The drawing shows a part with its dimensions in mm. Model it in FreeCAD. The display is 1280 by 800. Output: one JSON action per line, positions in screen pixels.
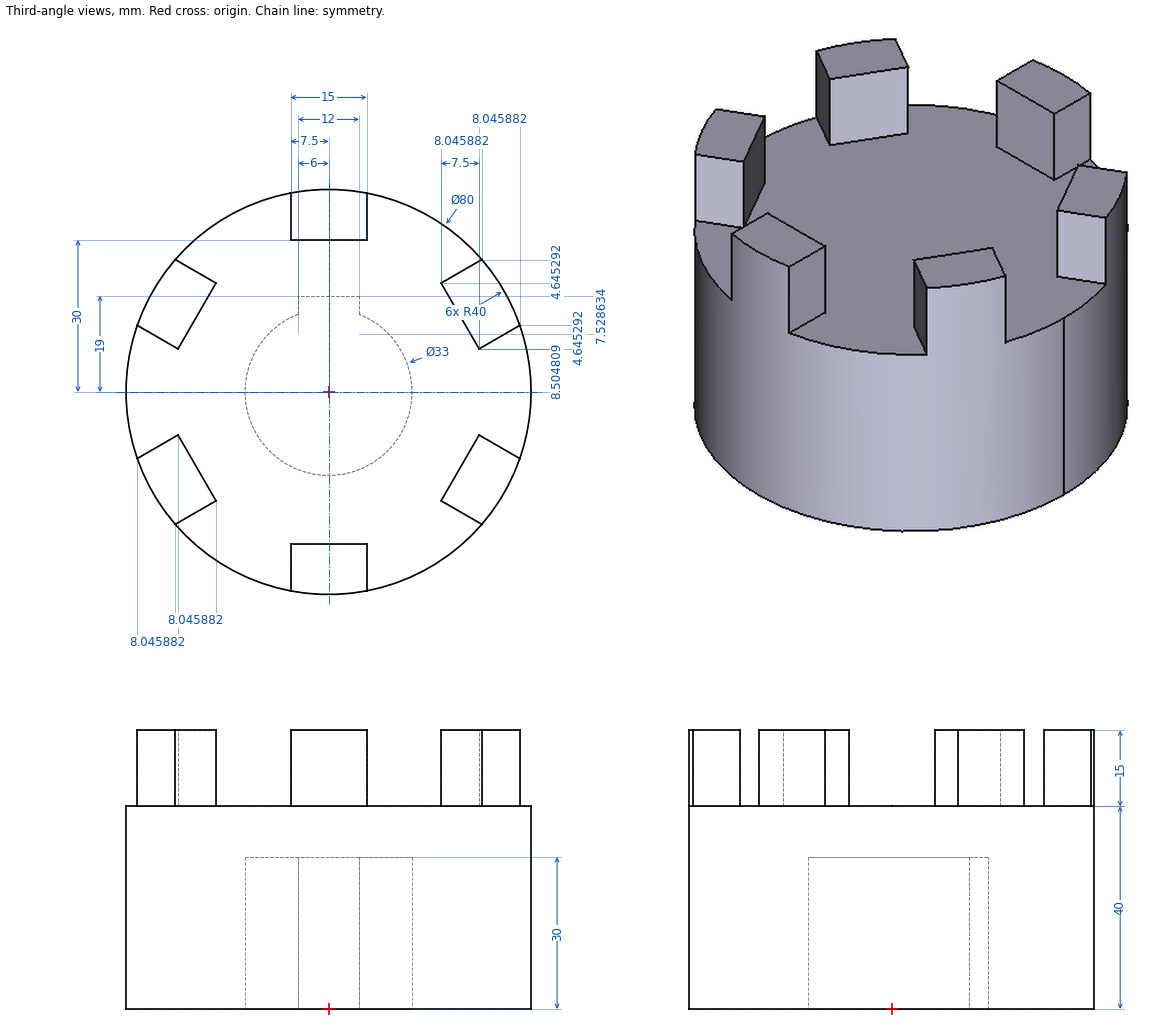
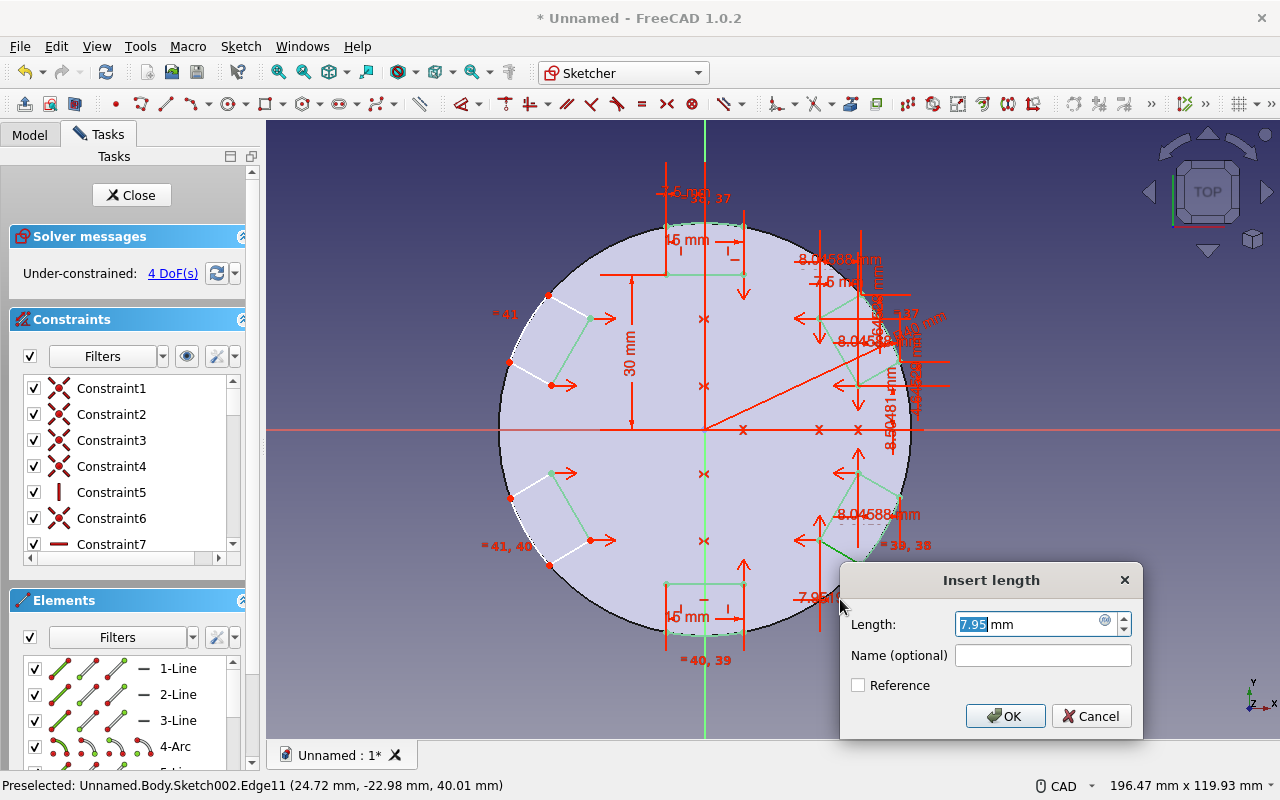
{"action": "type", "text": "8.045882"}
{"action": "key", "text": "Return"}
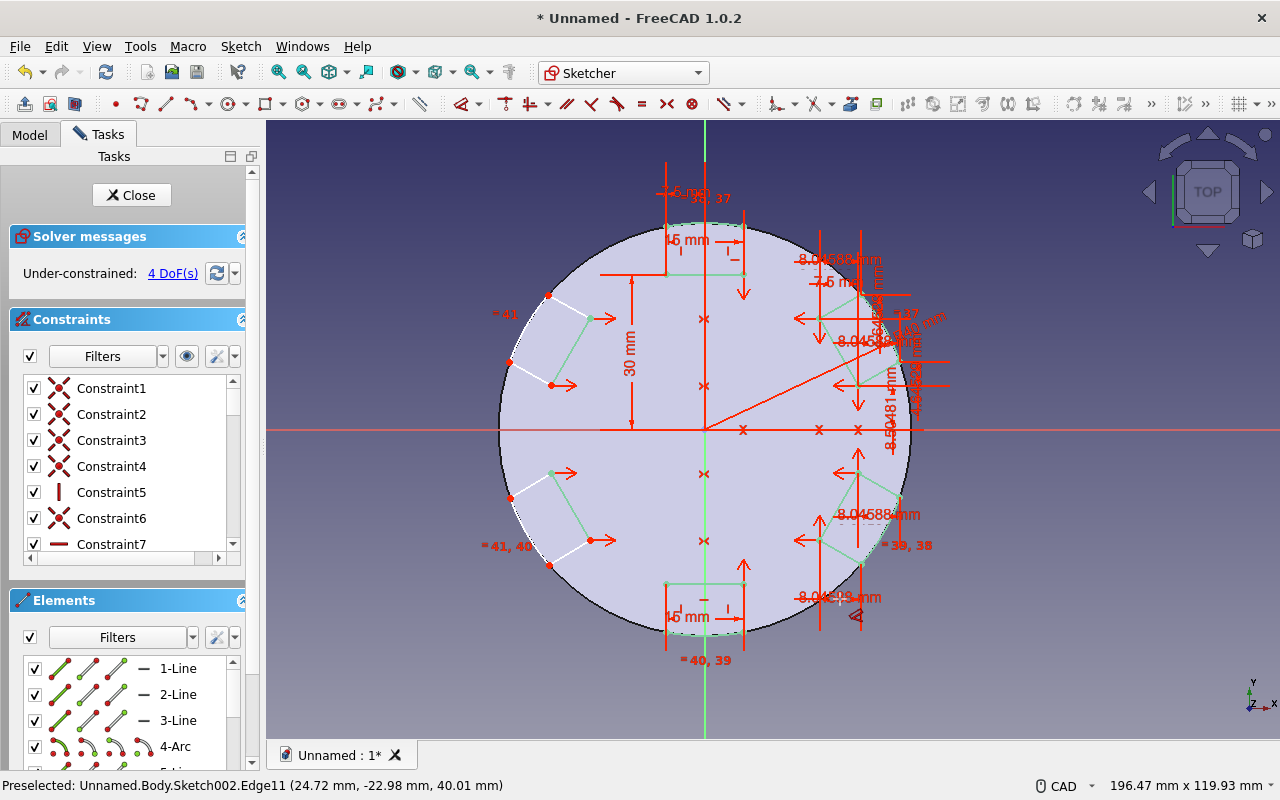
{"action": "left_click", "coordinate": [562, 558]}
{"action": "left_click", "coordinate": [570, 599]}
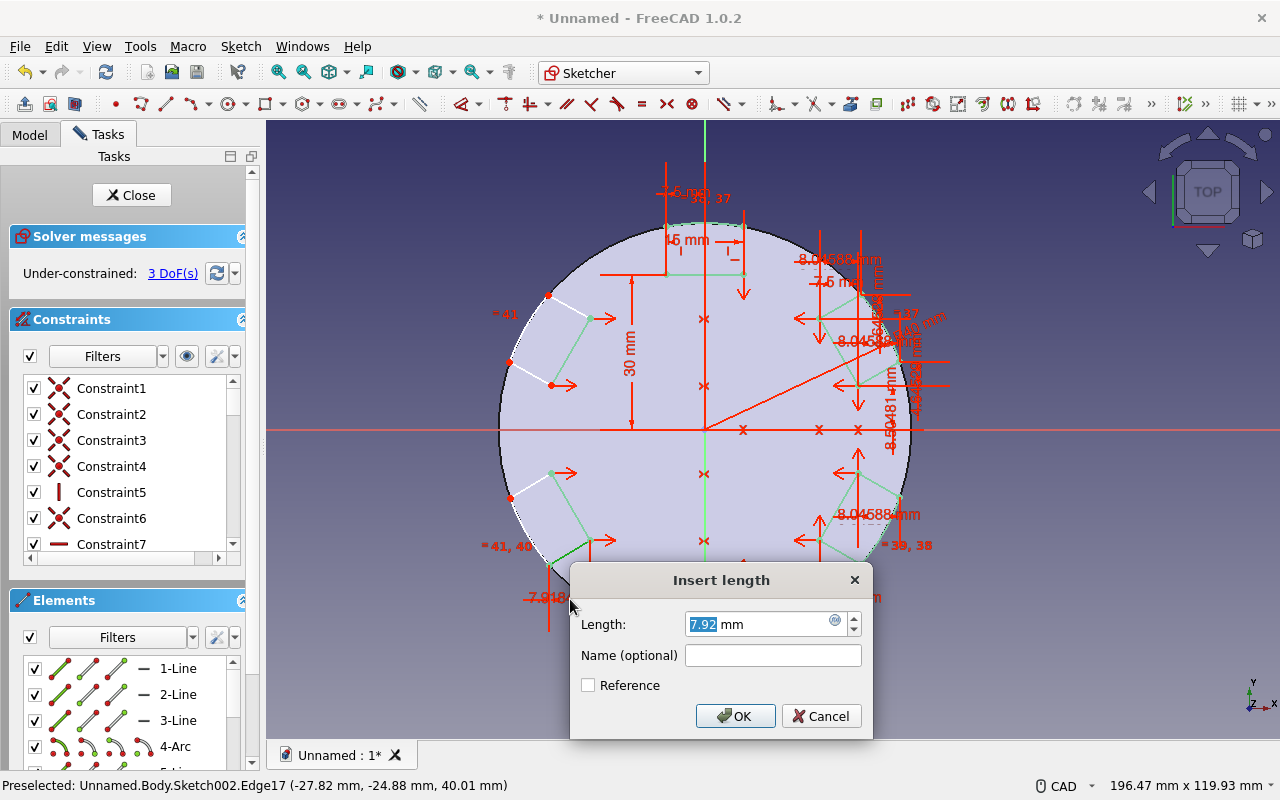
{"action": "type", "text": "8.045882"}
{"action": "key", "text": "Return"}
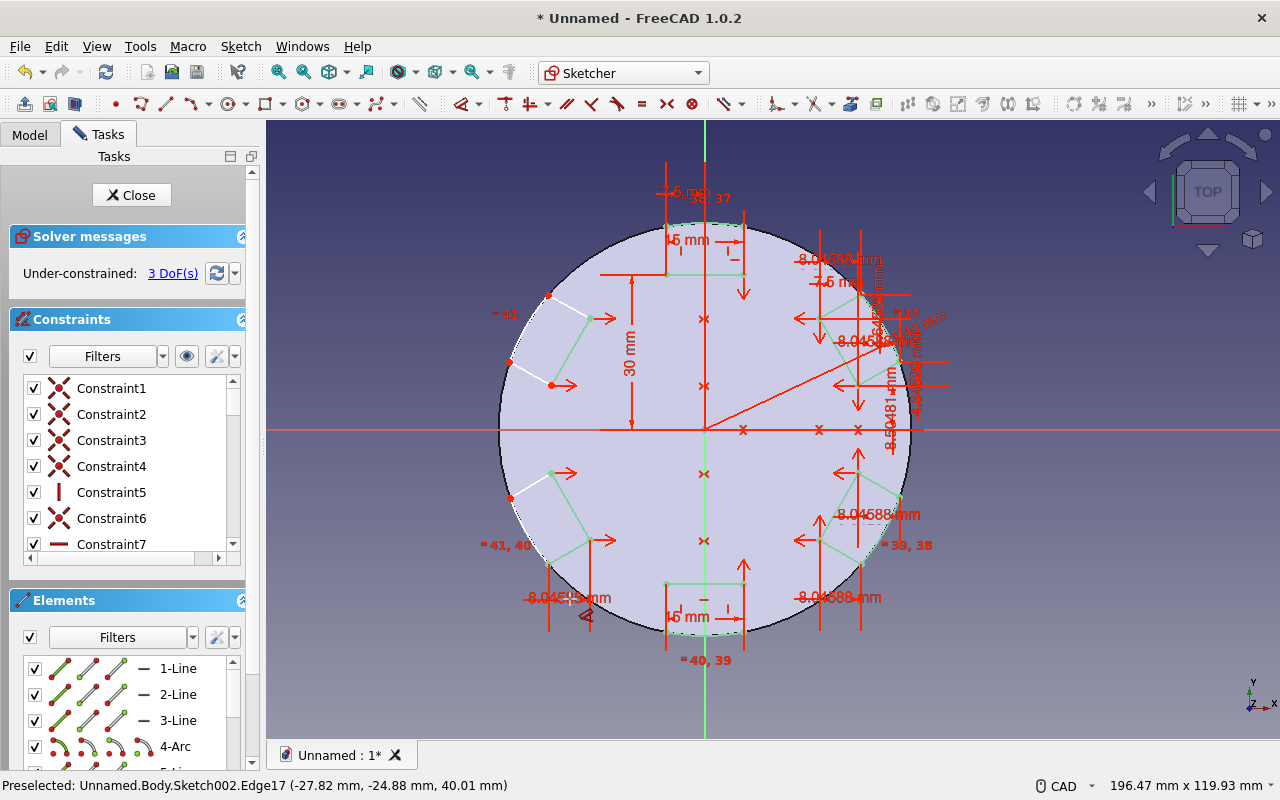
{"action": "left_click", "coordinate": [539, 481]}
{"action": "left_click", "coordinate": [545, 532]}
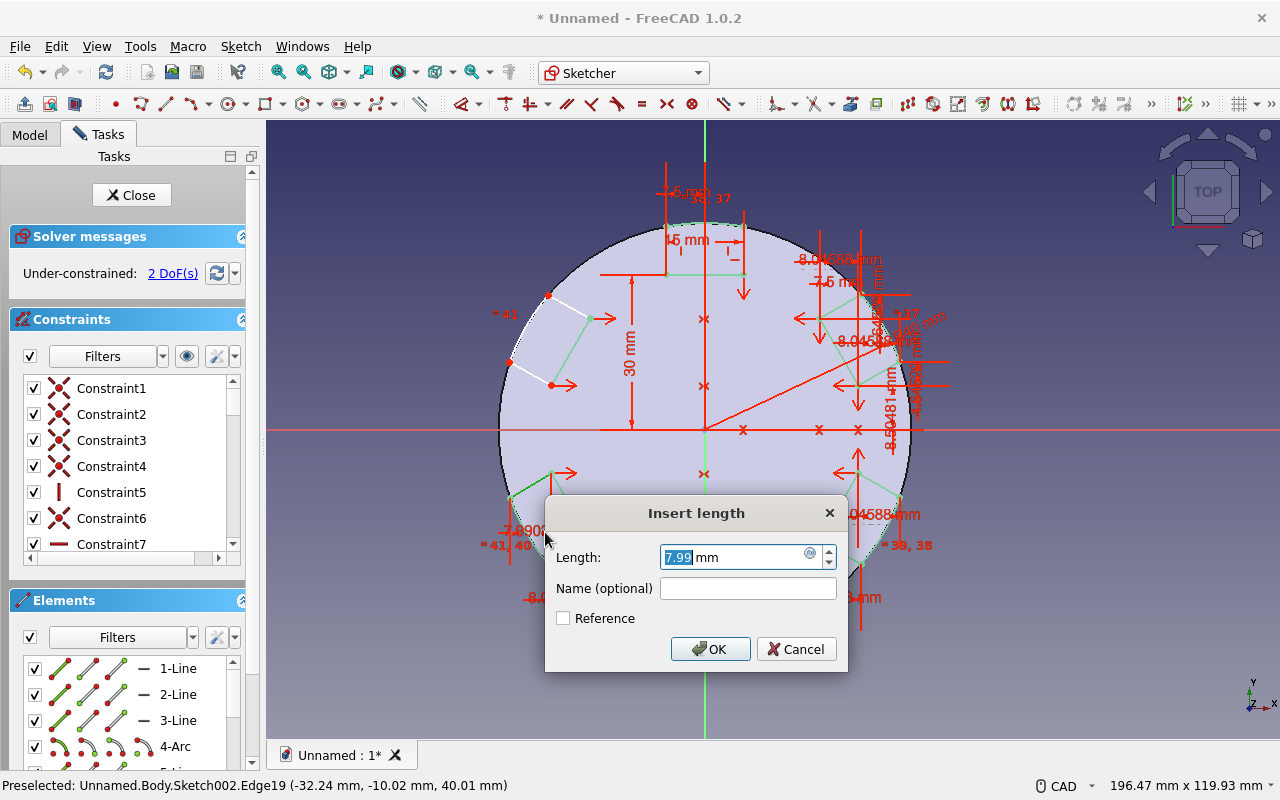
{"action": "type", "text": "8.045882"}
{"action": "key", "text": "Return"}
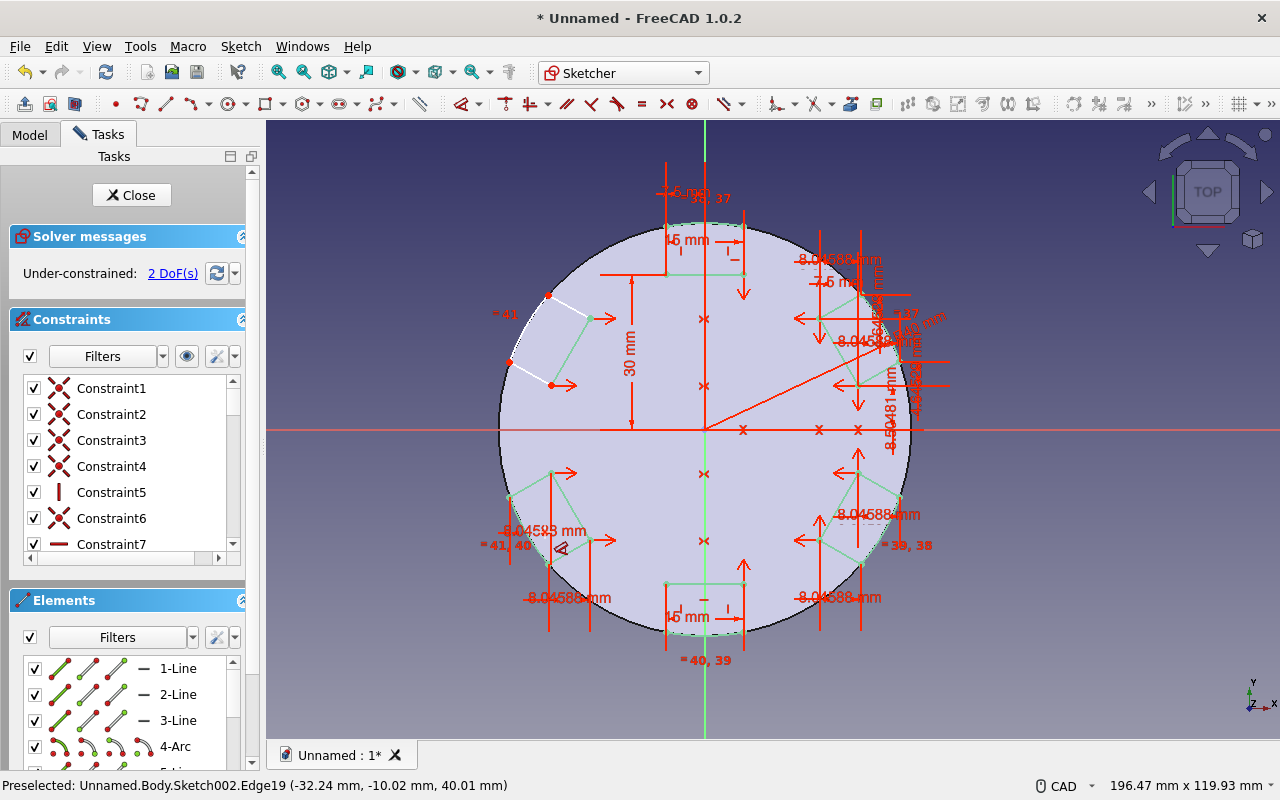
{"action": "left_click", "coordinate": [522, 369]}
{"action": "left_click", "coordinate": [540, 328]}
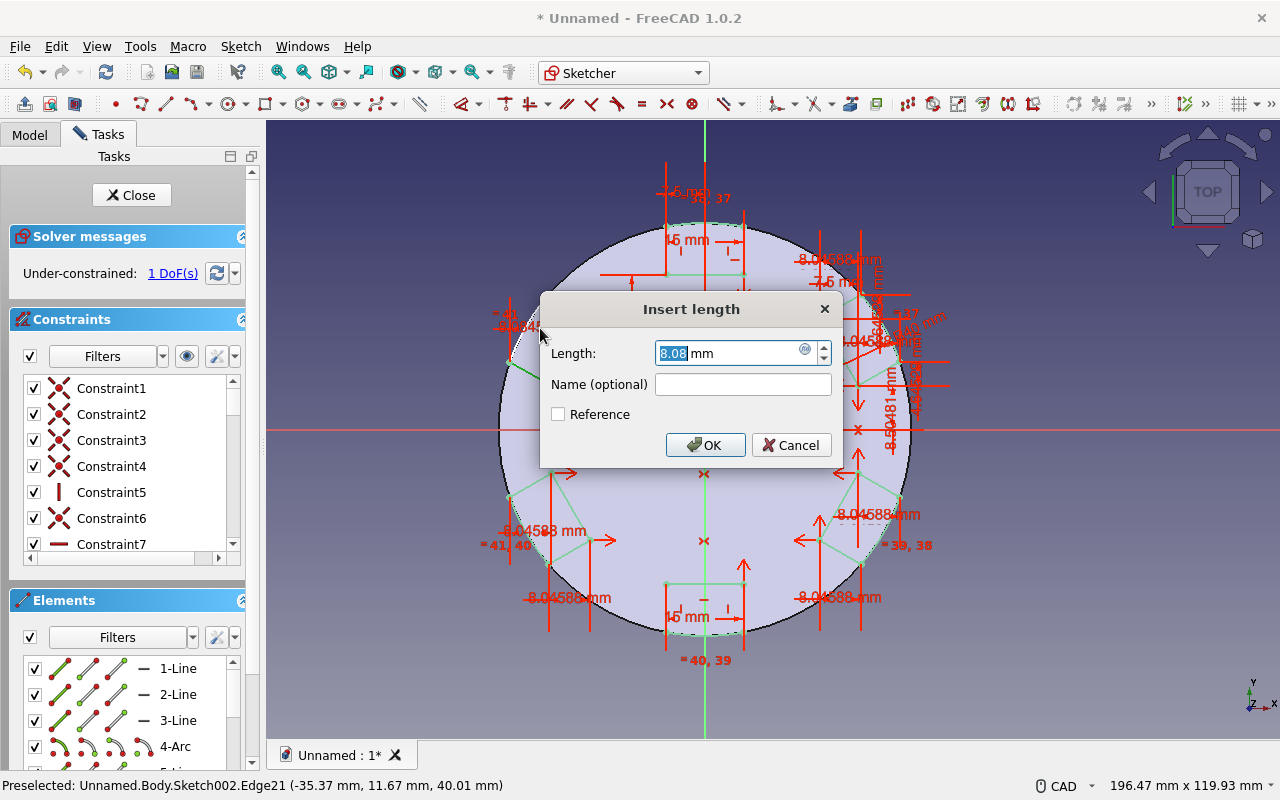
{"action": "type", "text": "8.045882"}
{"action": "key", "text": "Return"}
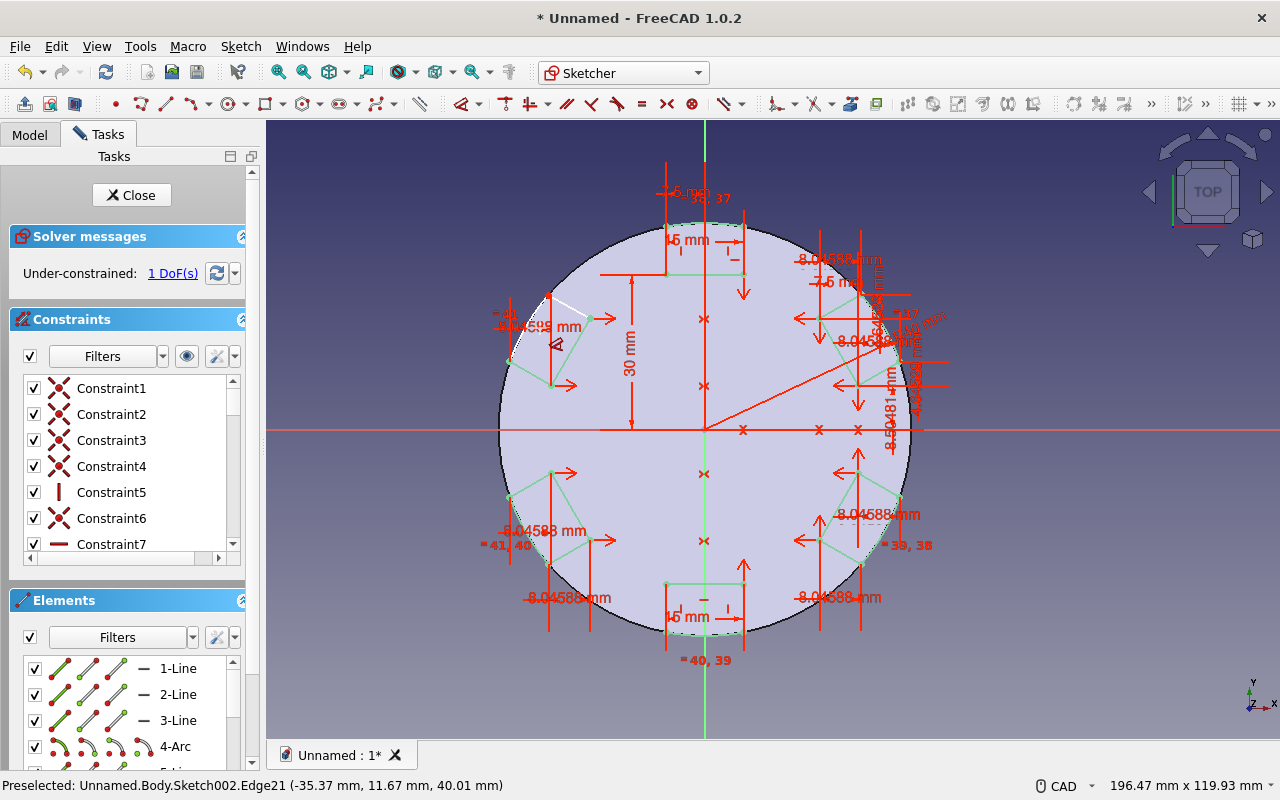
{"action": "left_click", "coordinate": [578, 312]}
{"action": "left_click", "coordinate": [569, 261]}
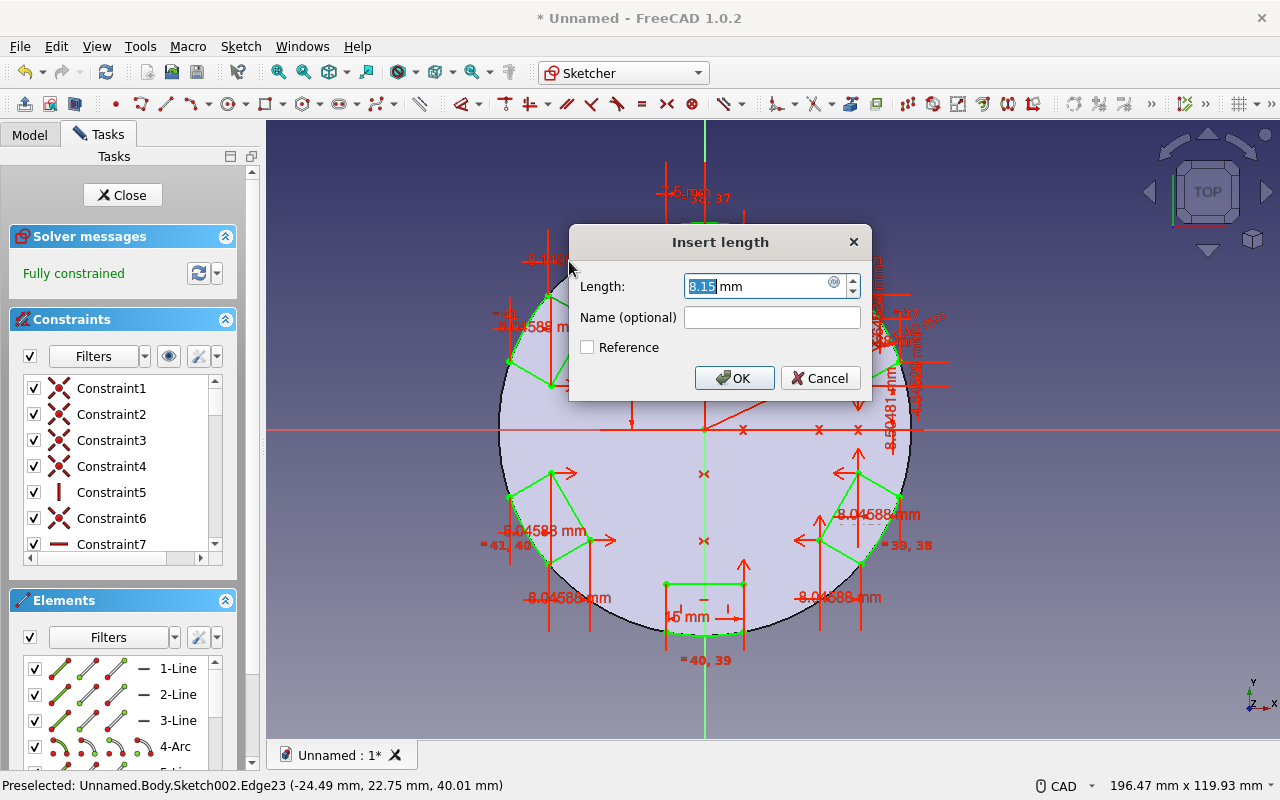
{"action": "type", "text": "8.045882"}
{"action": "key", "text": "Return"}
{"action": "key", "text": "Escape"}